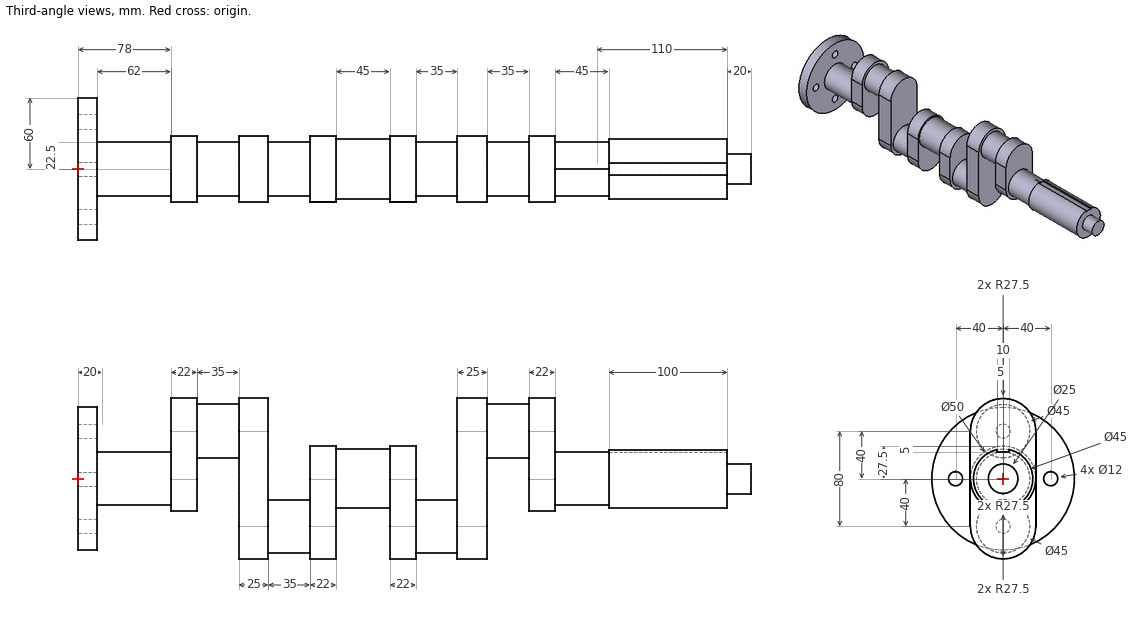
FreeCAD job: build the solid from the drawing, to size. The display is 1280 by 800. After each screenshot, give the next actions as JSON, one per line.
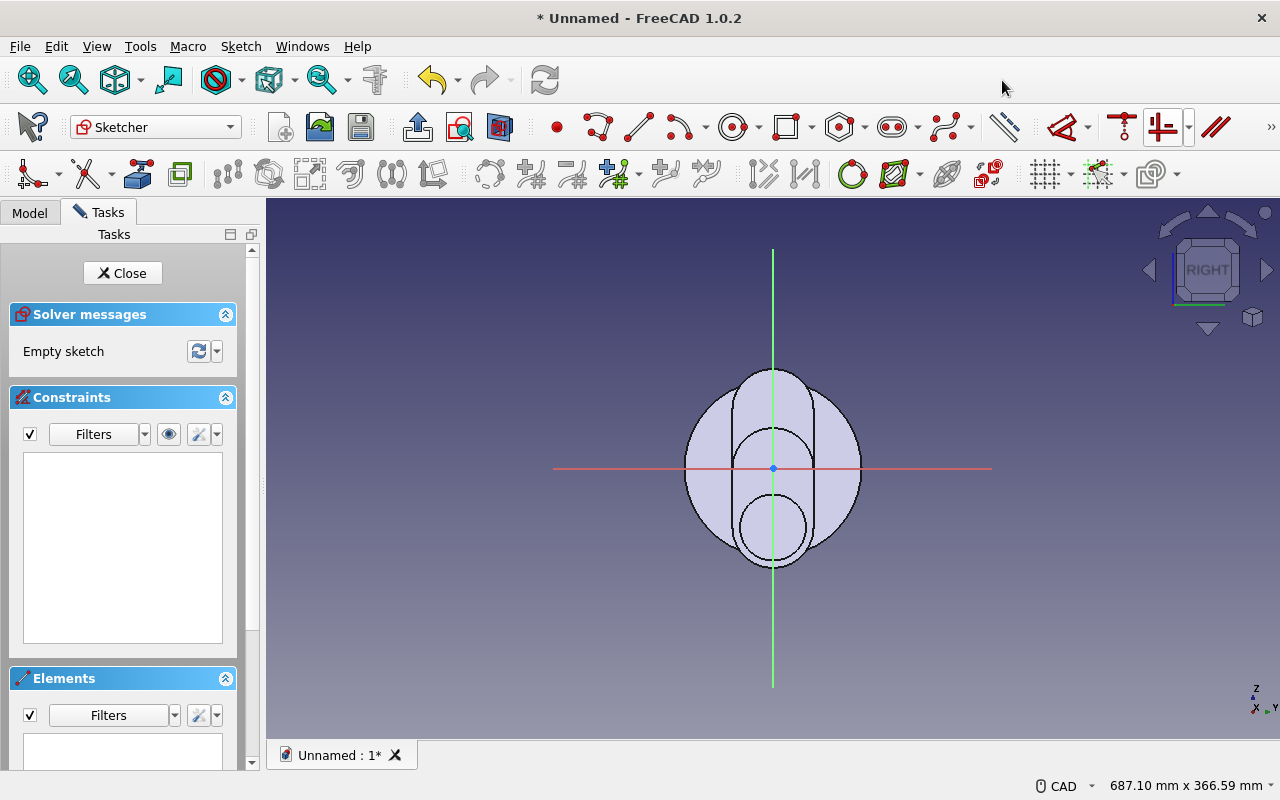
{"action": "scroll", "coordinate": [856, 468], "scroll_direction": "up", "scroll_amount": 3}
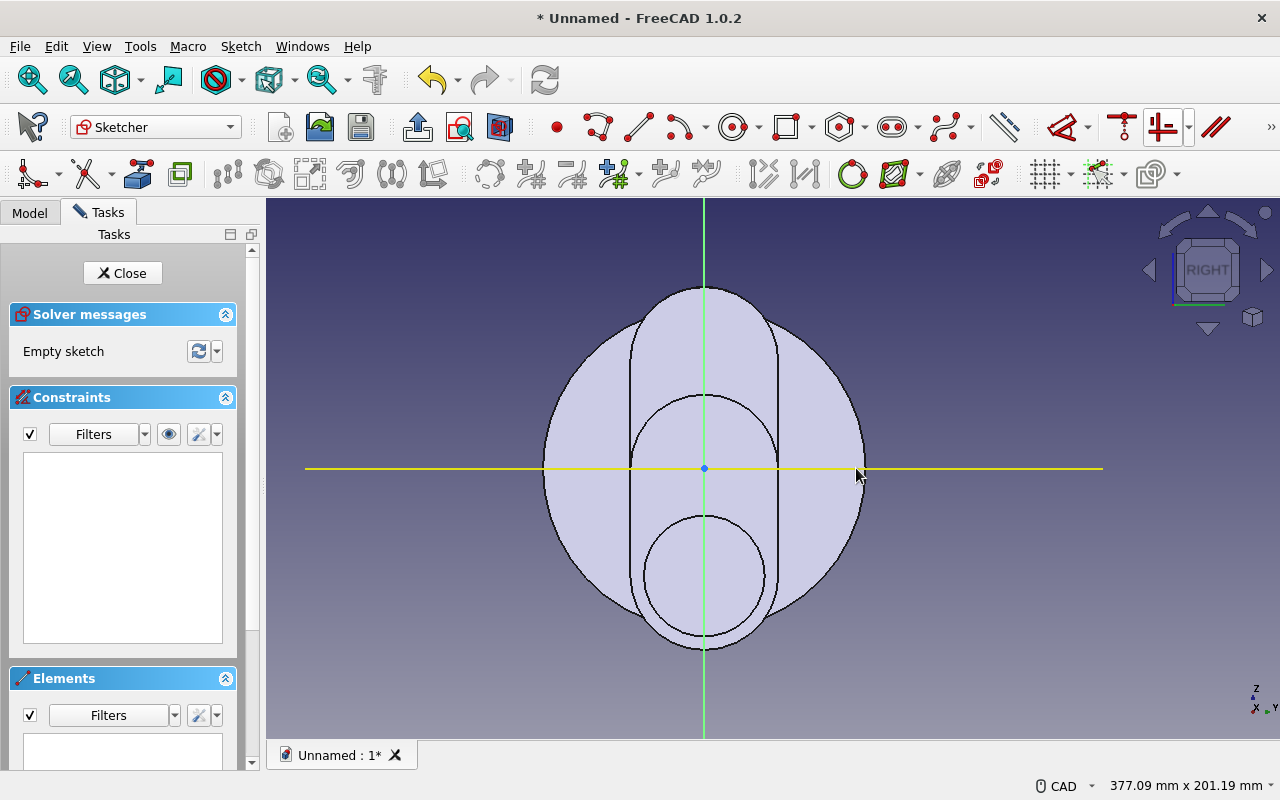
{"action": "left_click", "coordinate": [892, 128]}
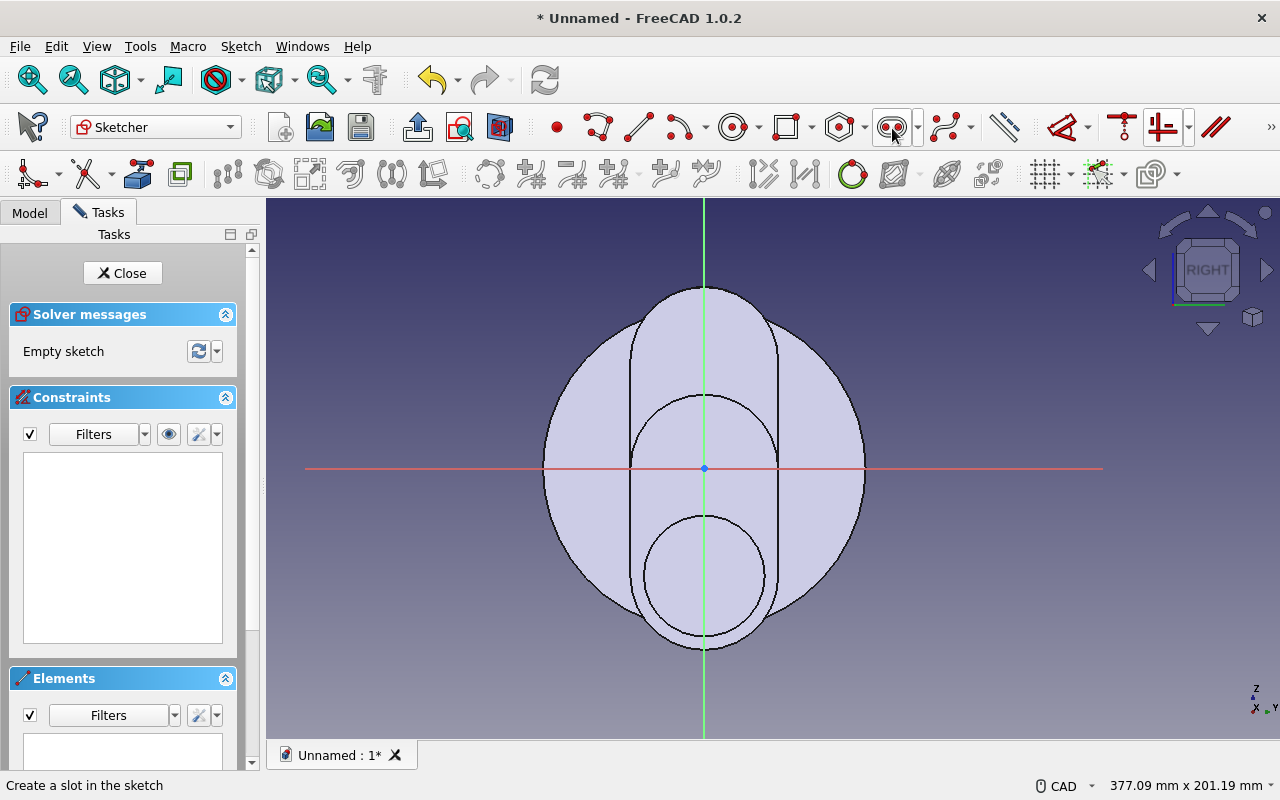
{"action": "left_click", "coordinate": [704, 576]}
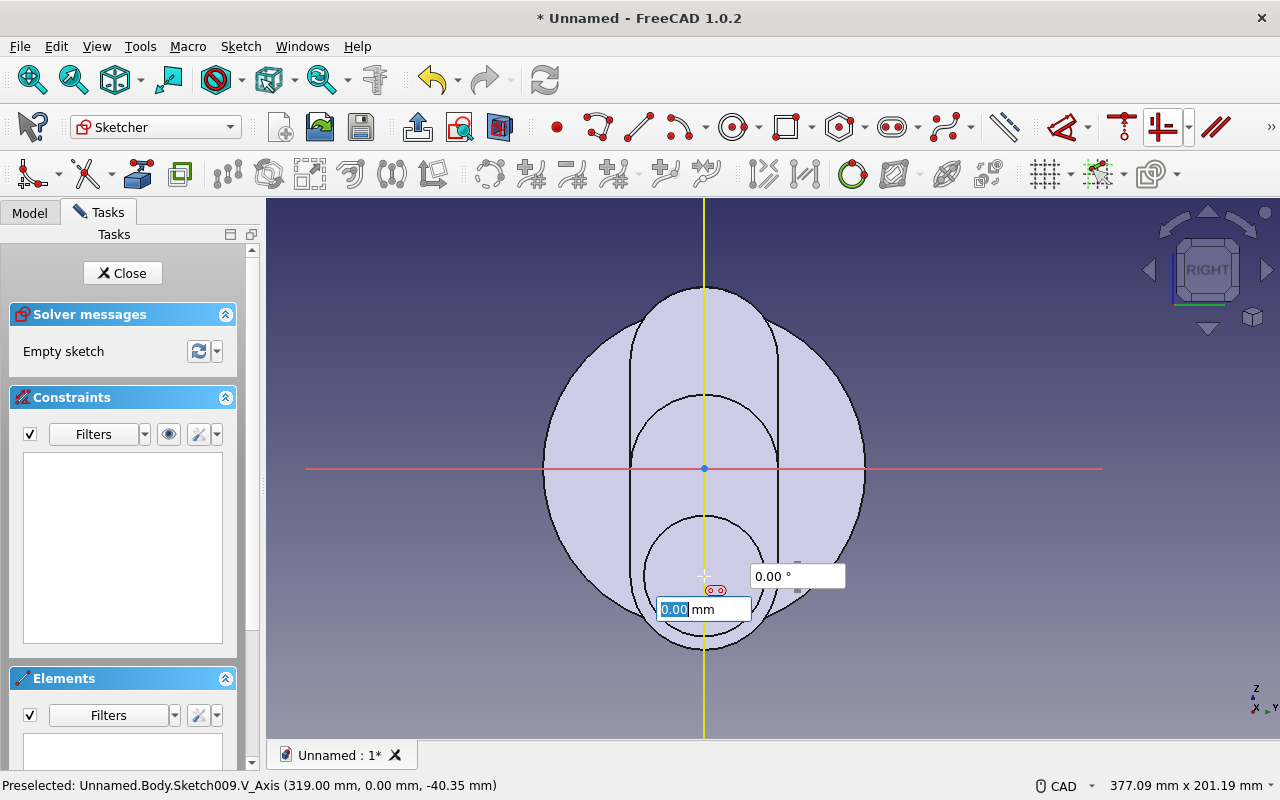
{"action": "left_click", "coordinate": [713, 361]}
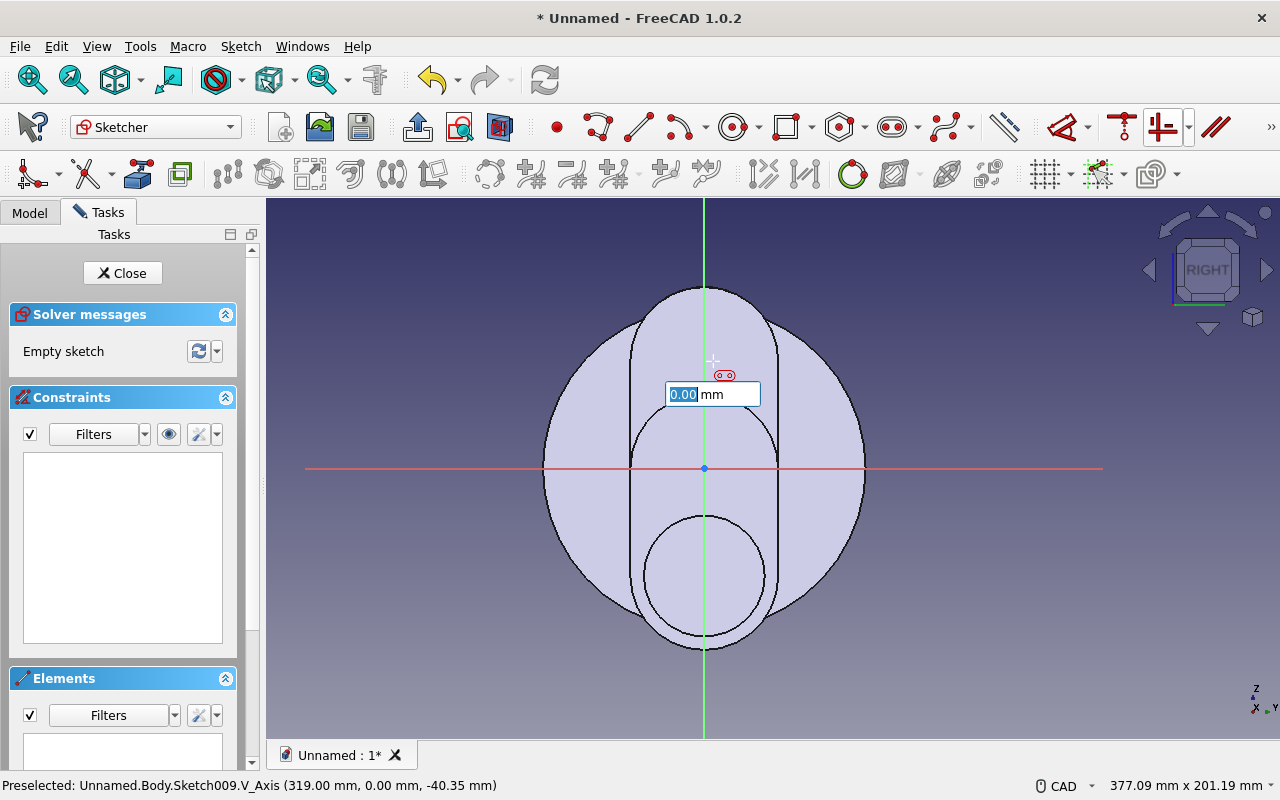
{"action": "left_click", "coordinate": [630, 436]}
{"action": "key", "text": "Escape"}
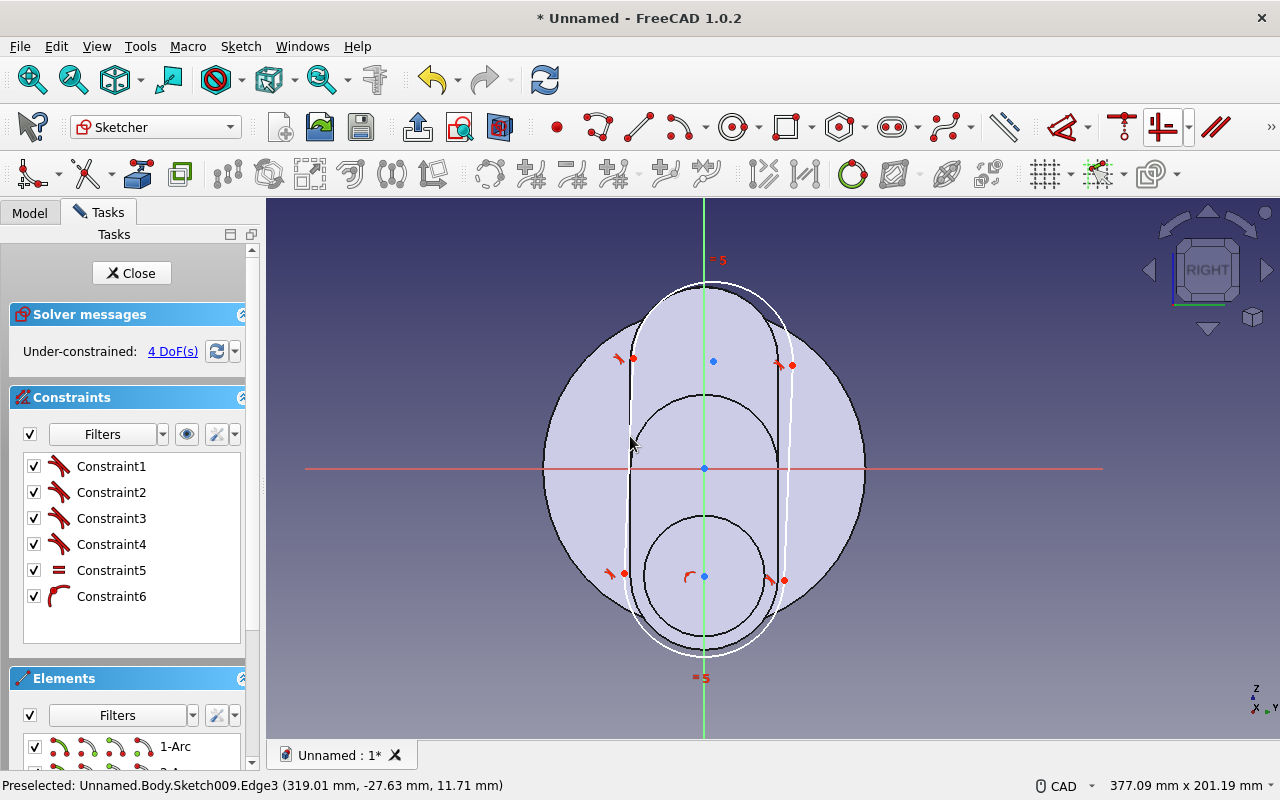
{"action": "left_click", "coordinate": [627, 509]}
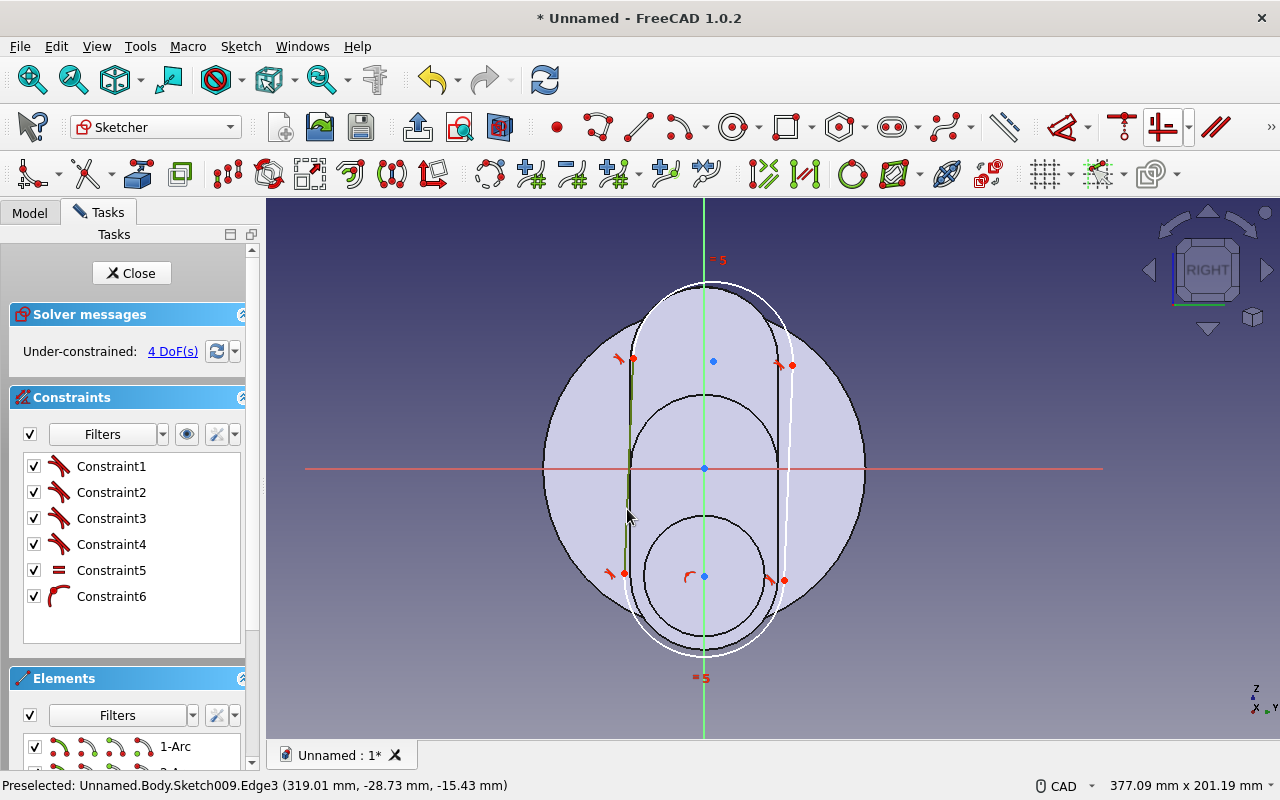
{"action": "key", "text": "v"}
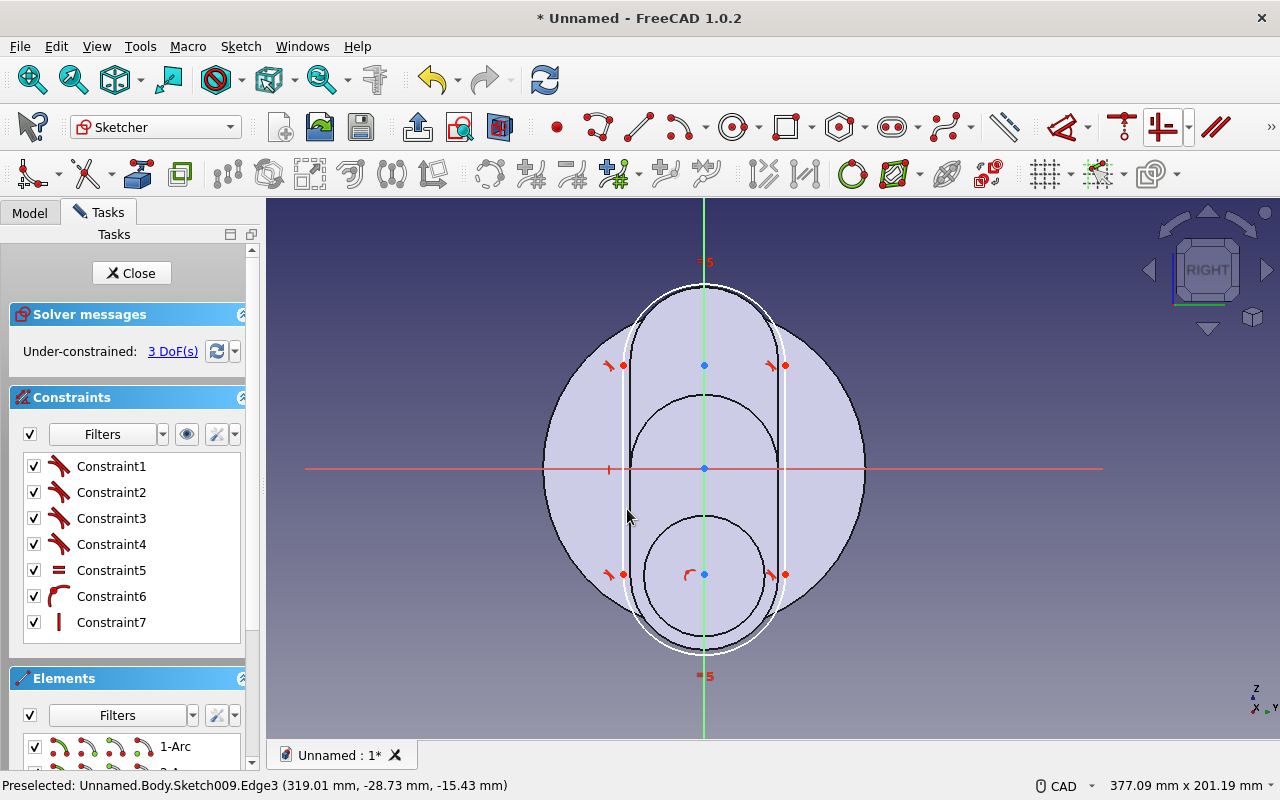
{"action": "left_click", "coordinate": [1062, 128]}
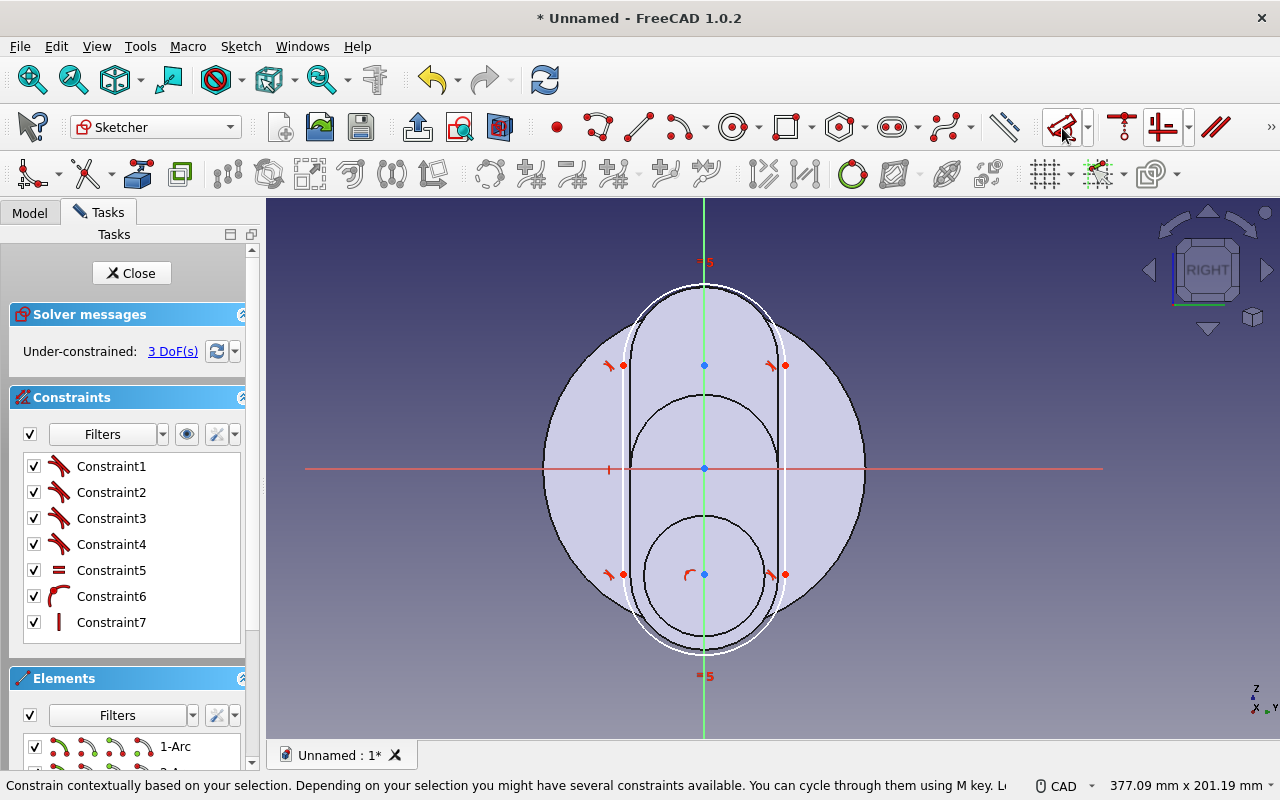
{"action": "left_click", "coordinate": [657, 640]}
{"action": "left_click", "coordinate": [638, 666]}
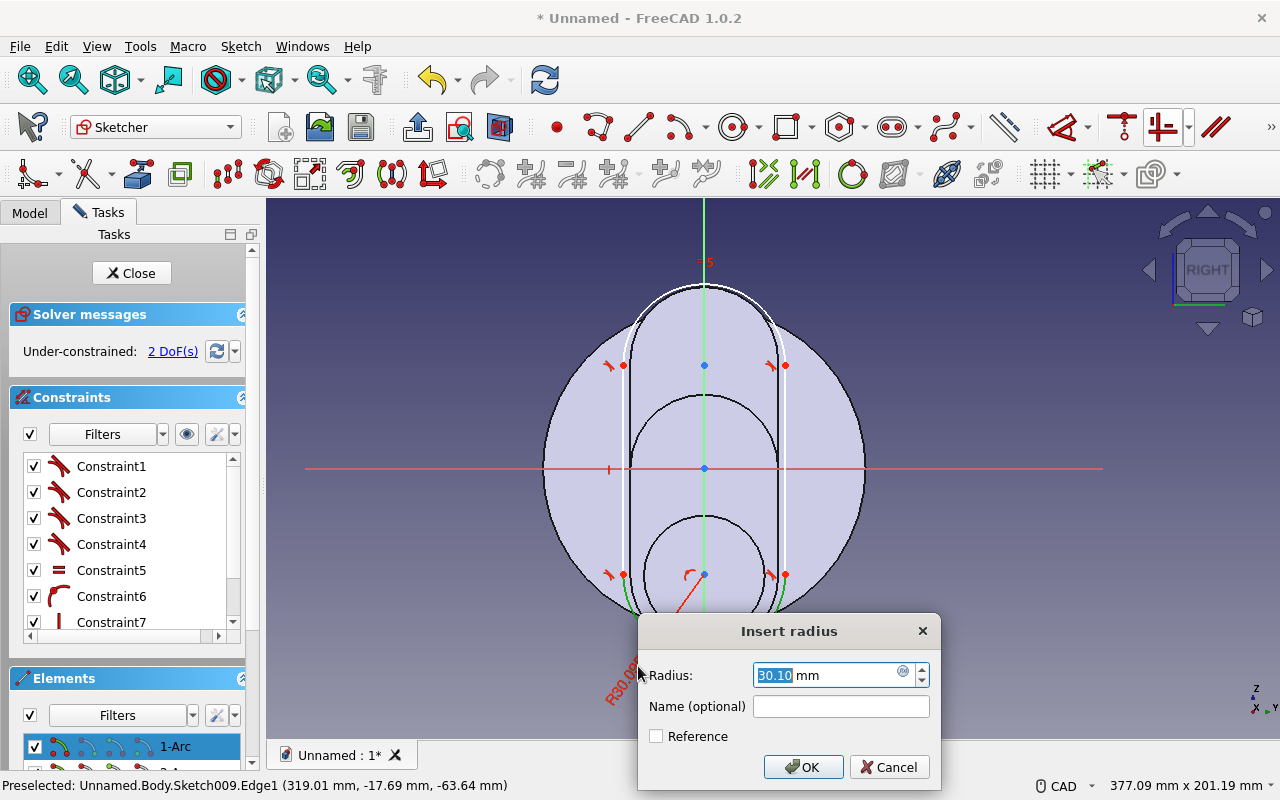
{"action": "type", "text": "27.5"}
{"action": "key", "text": "Return"}